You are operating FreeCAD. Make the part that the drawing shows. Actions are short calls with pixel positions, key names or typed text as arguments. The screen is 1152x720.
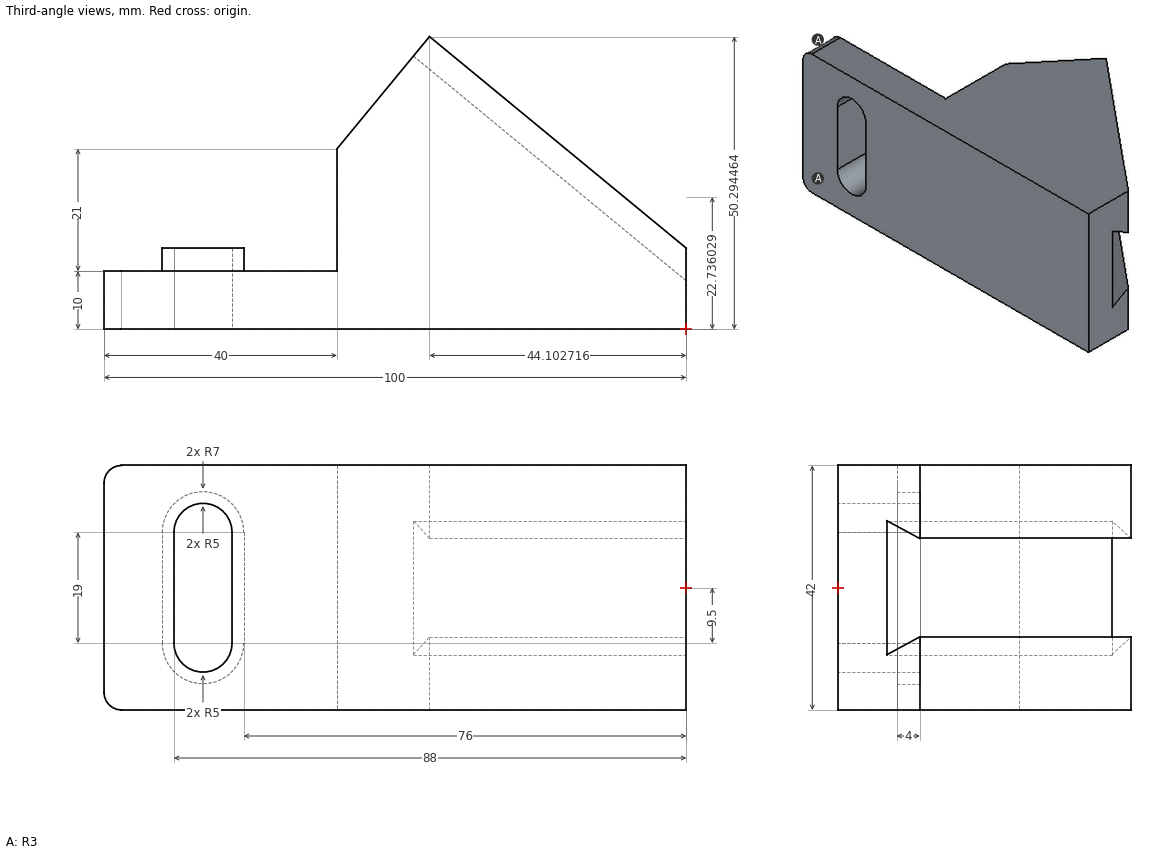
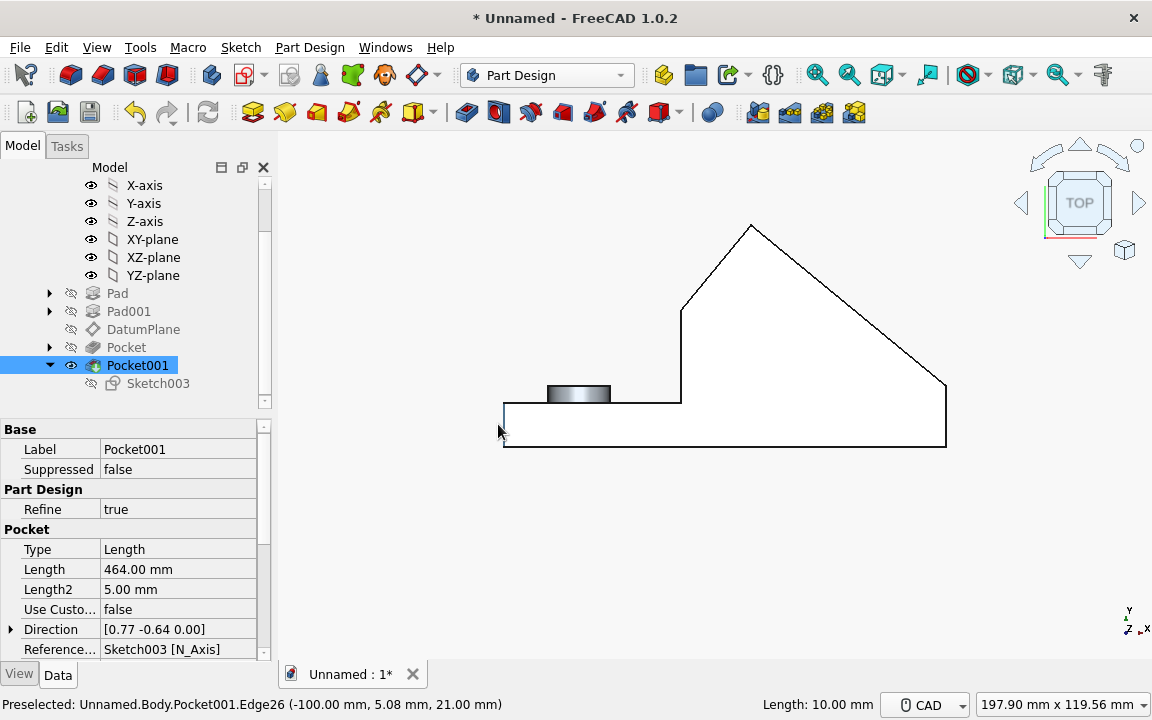
key(1)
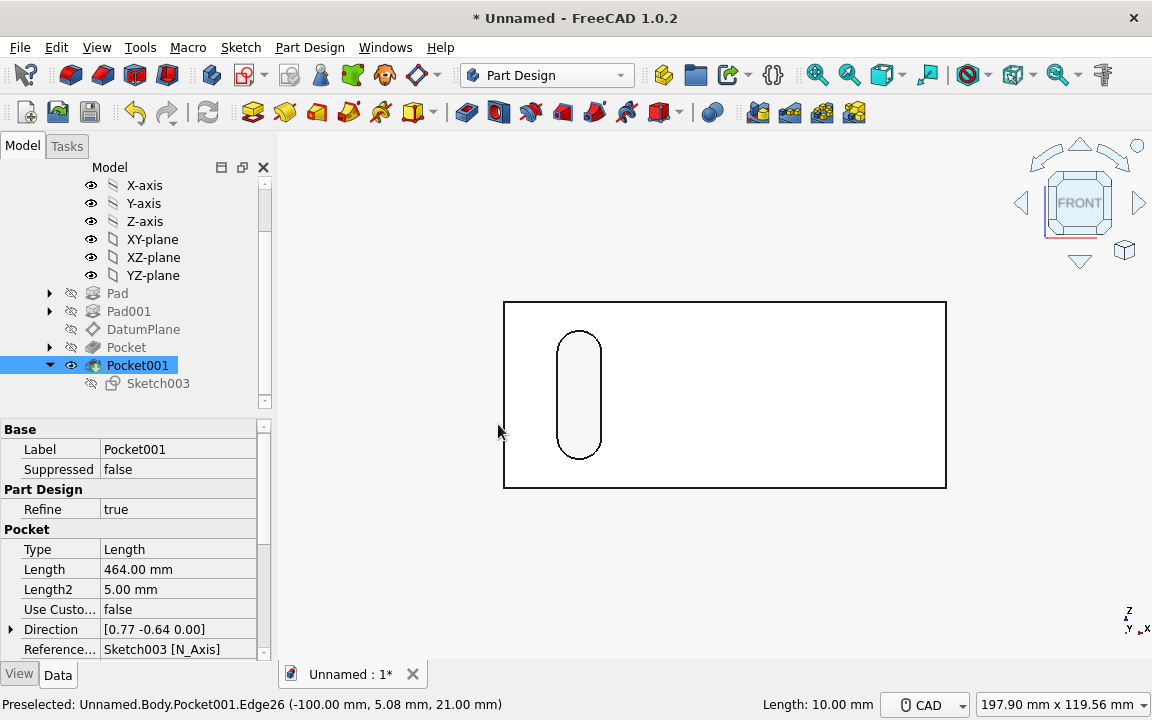
key(3)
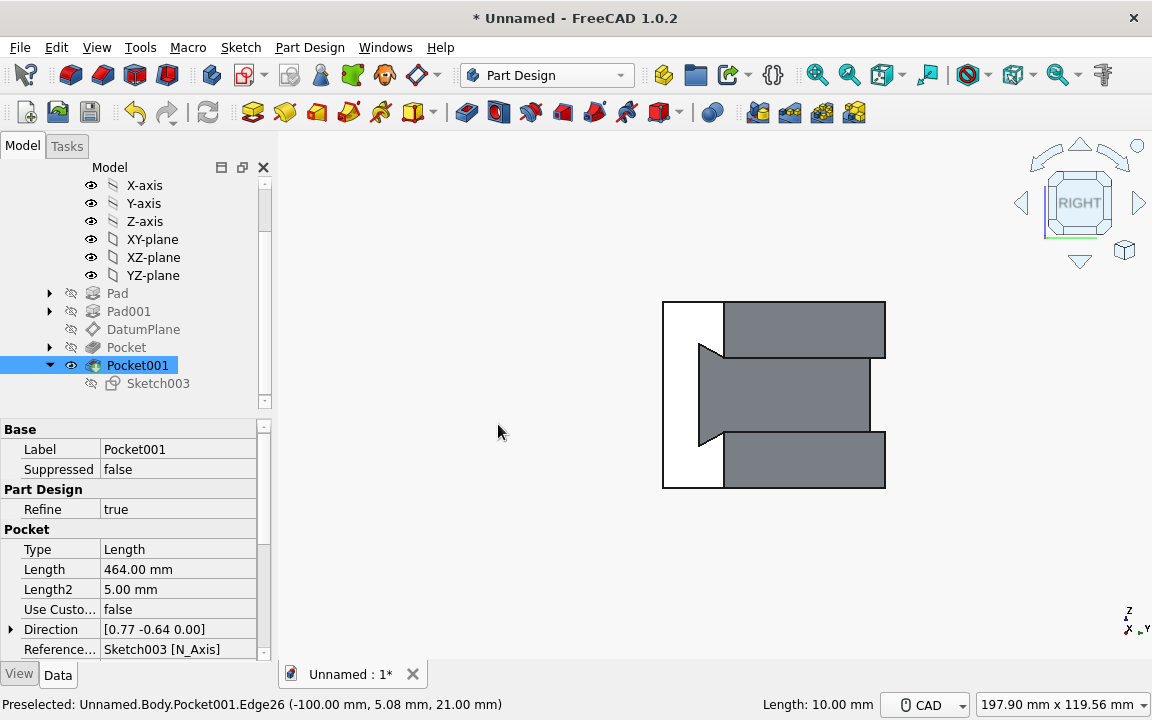
key(v)
key(f)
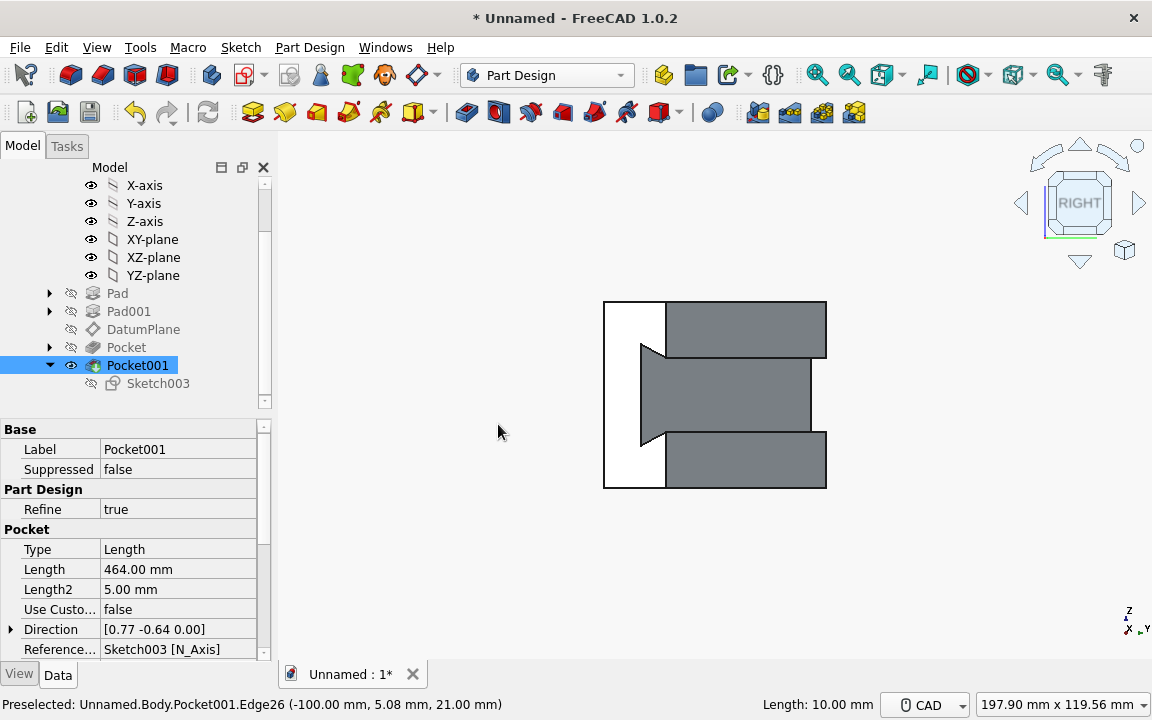
key(5)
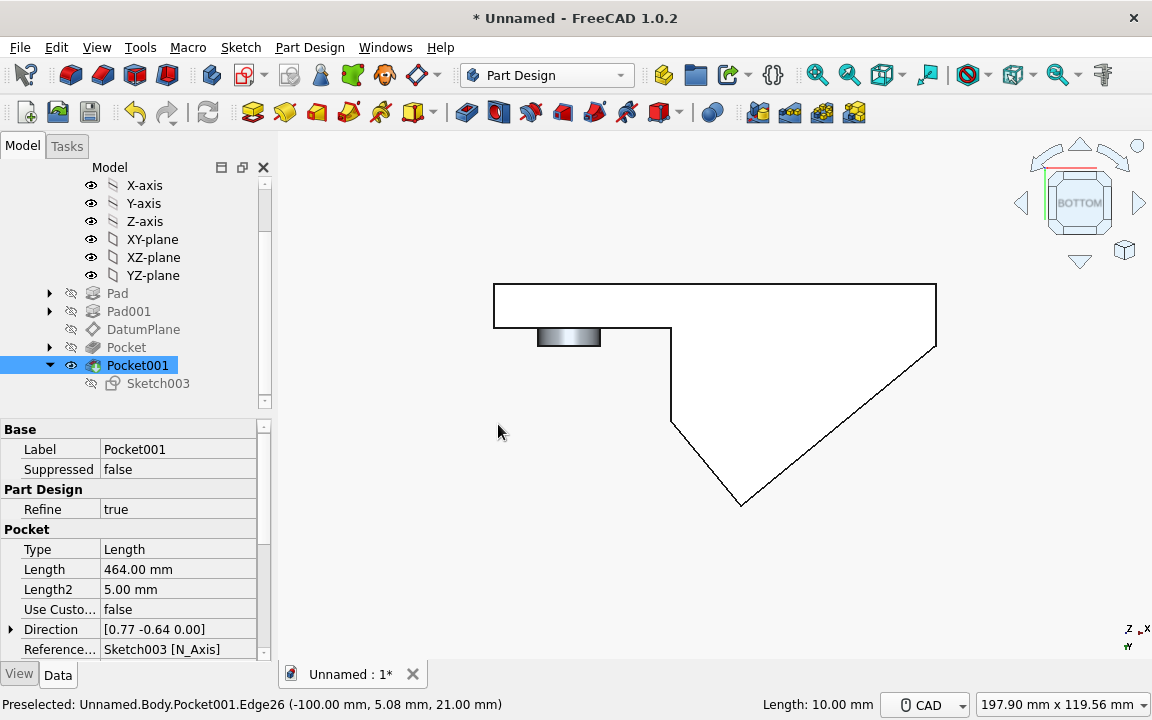
click(494, 305, ctrl)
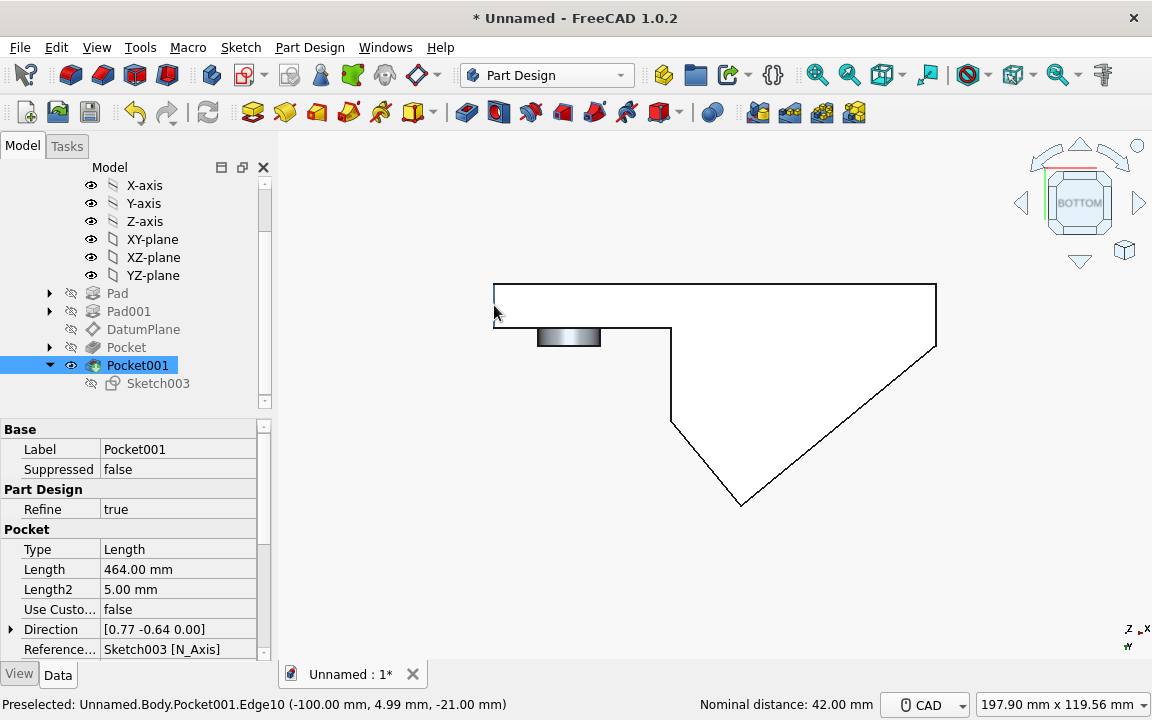
click(72, 76)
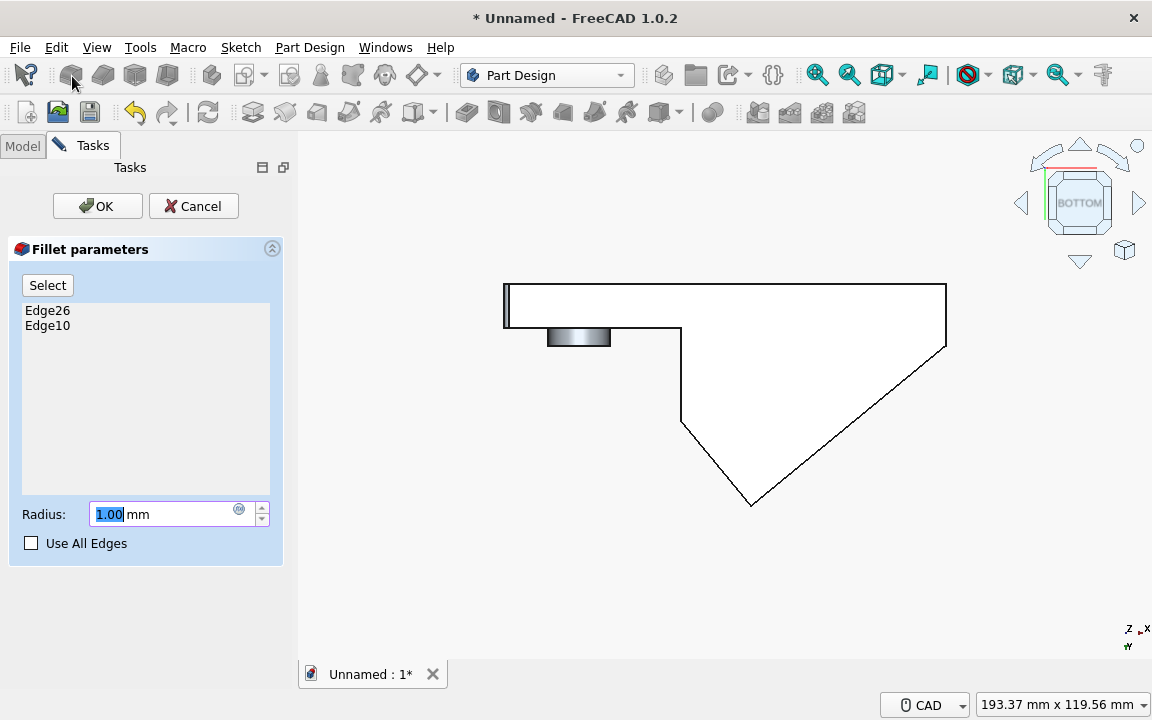
text(3)
key(Tab)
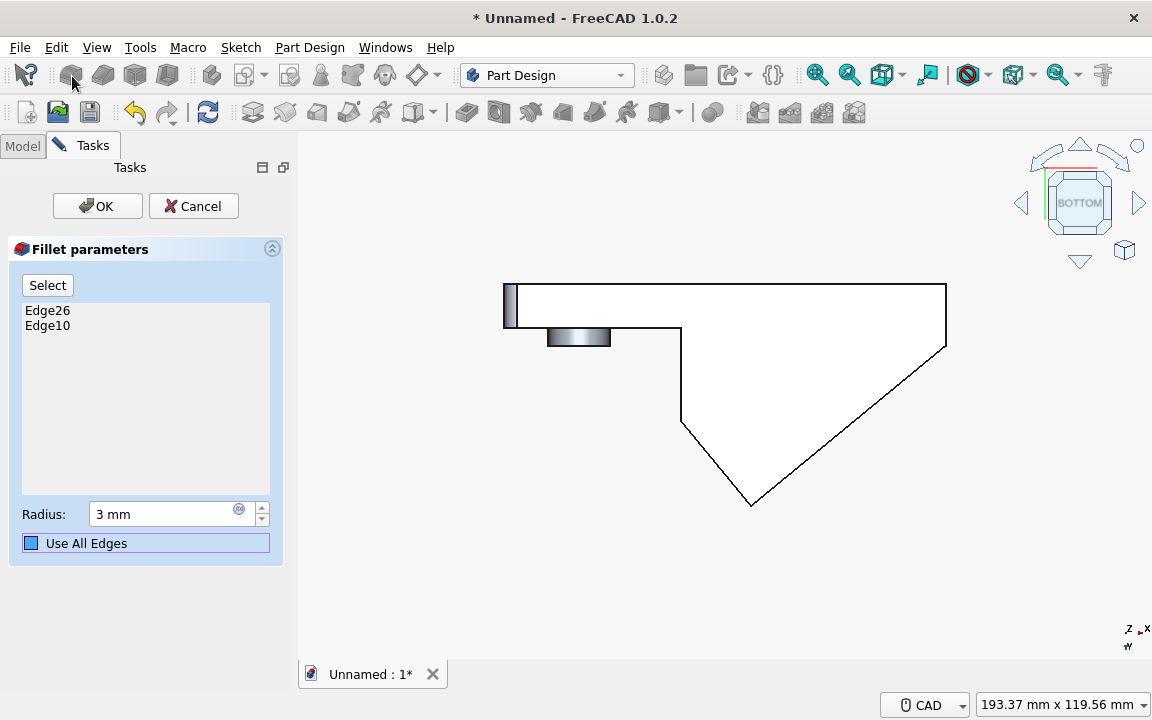
click(98, 206)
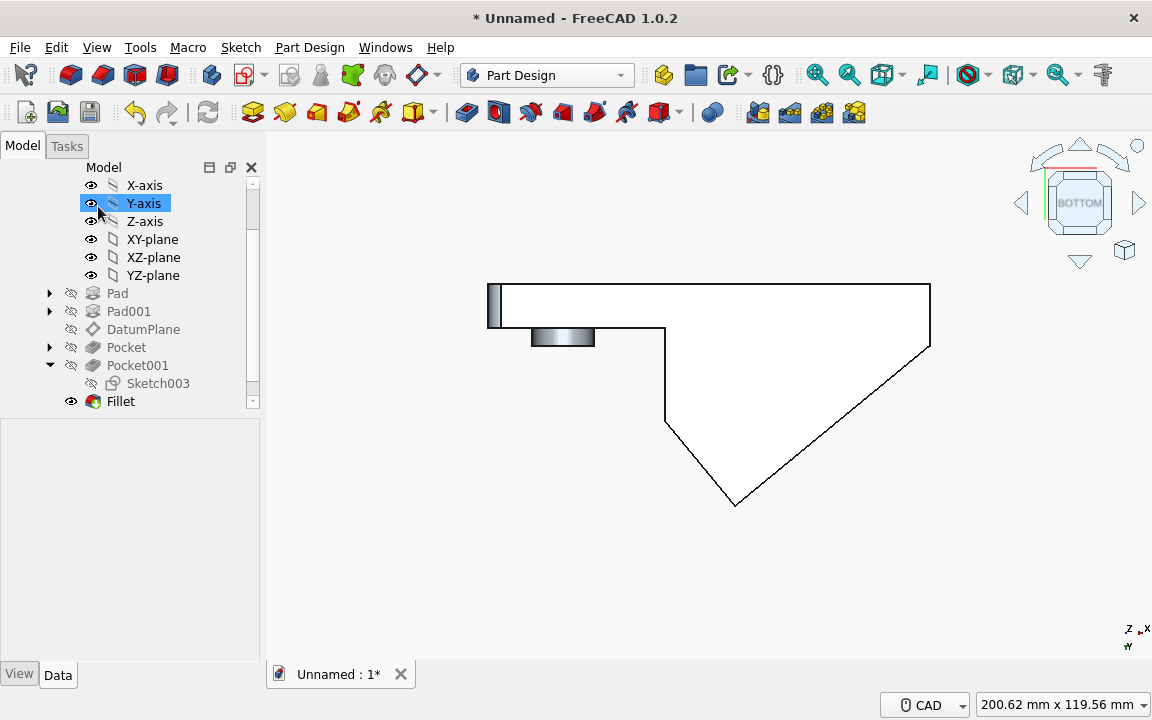
key(0)